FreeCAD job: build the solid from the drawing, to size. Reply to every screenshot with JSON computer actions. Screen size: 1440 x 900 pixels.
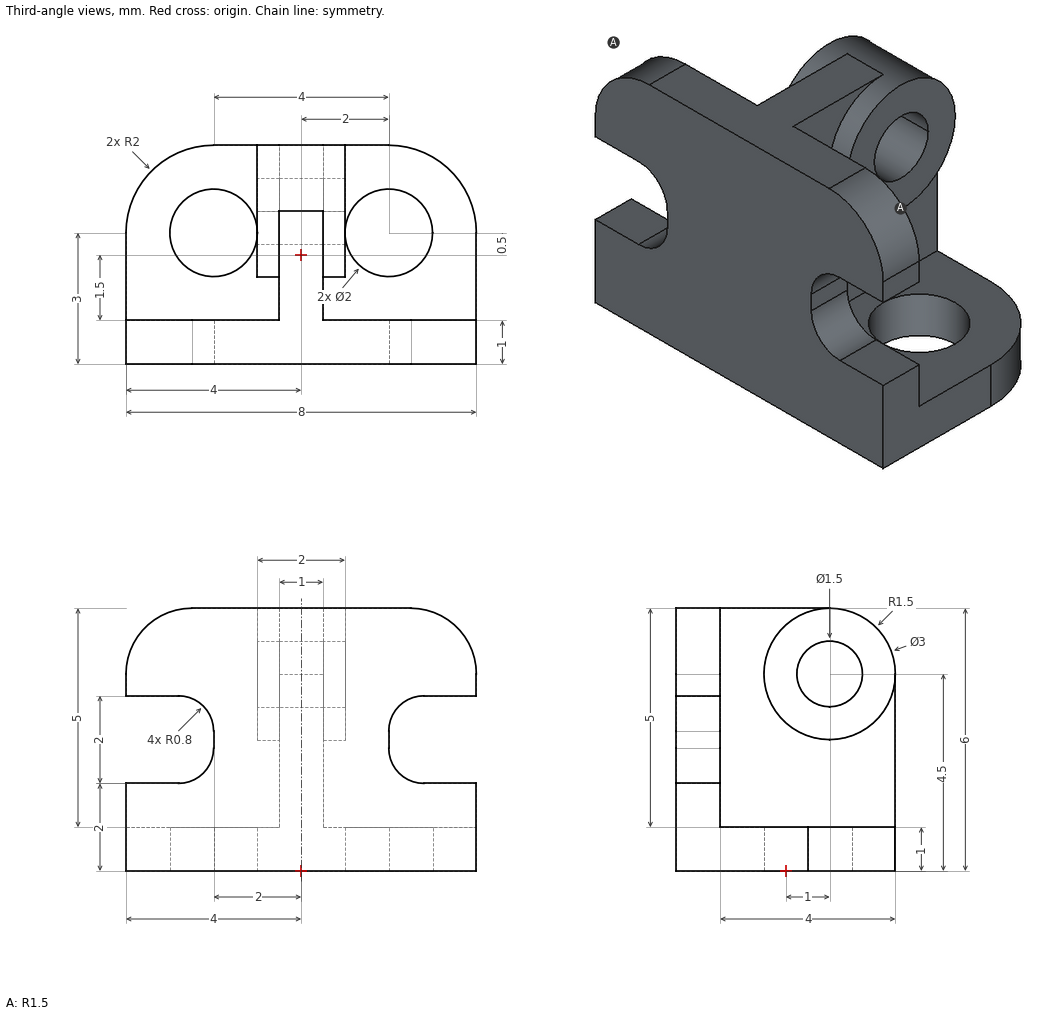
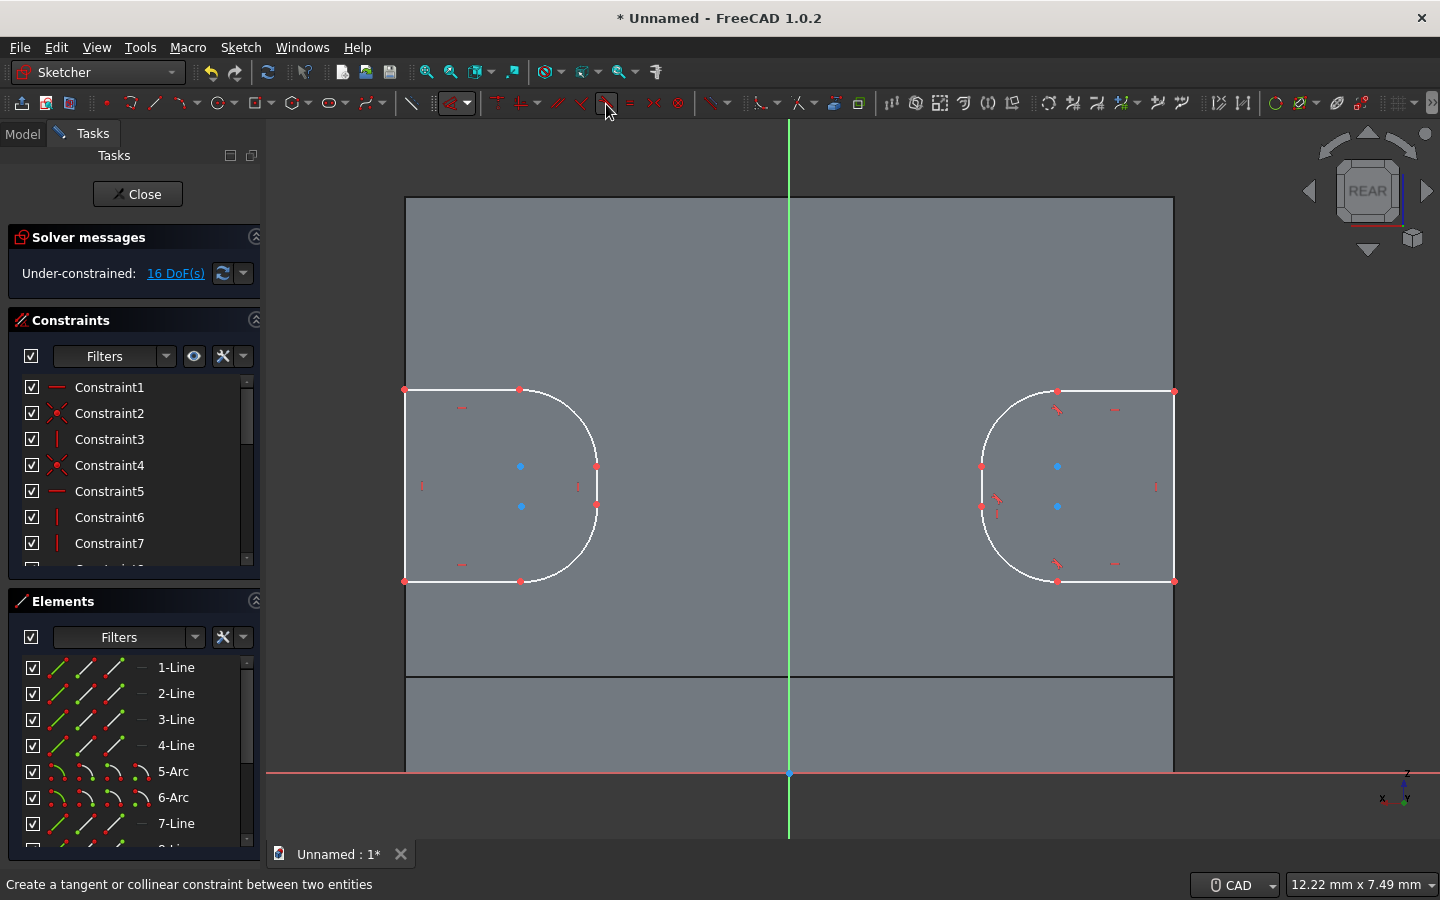
{"action": "left_click", "coordinate": [597, 494]}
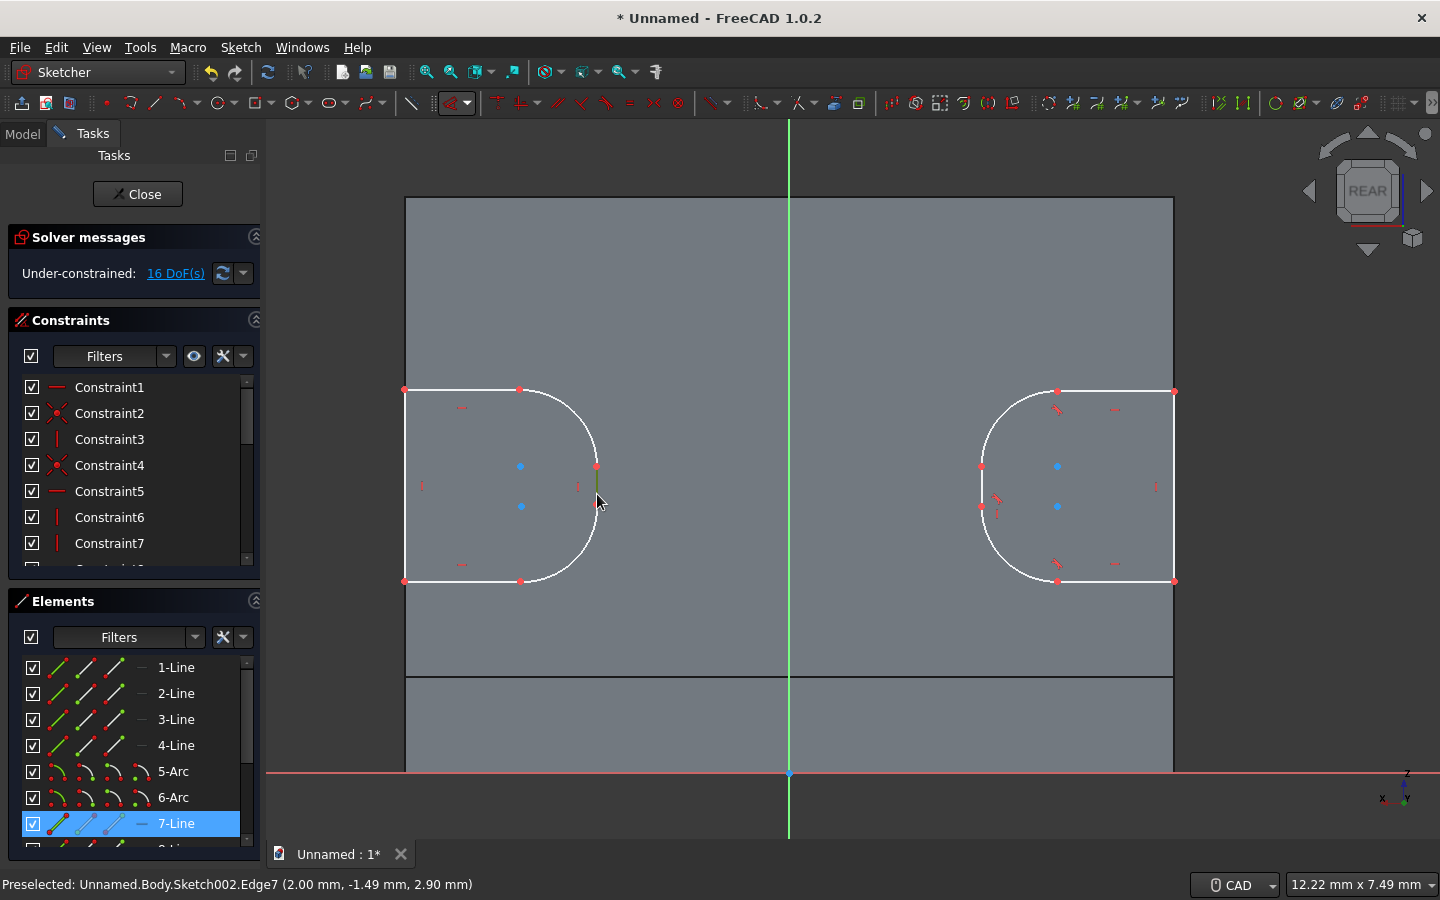
{"action": "left_click", "coordinate": [589, 432]}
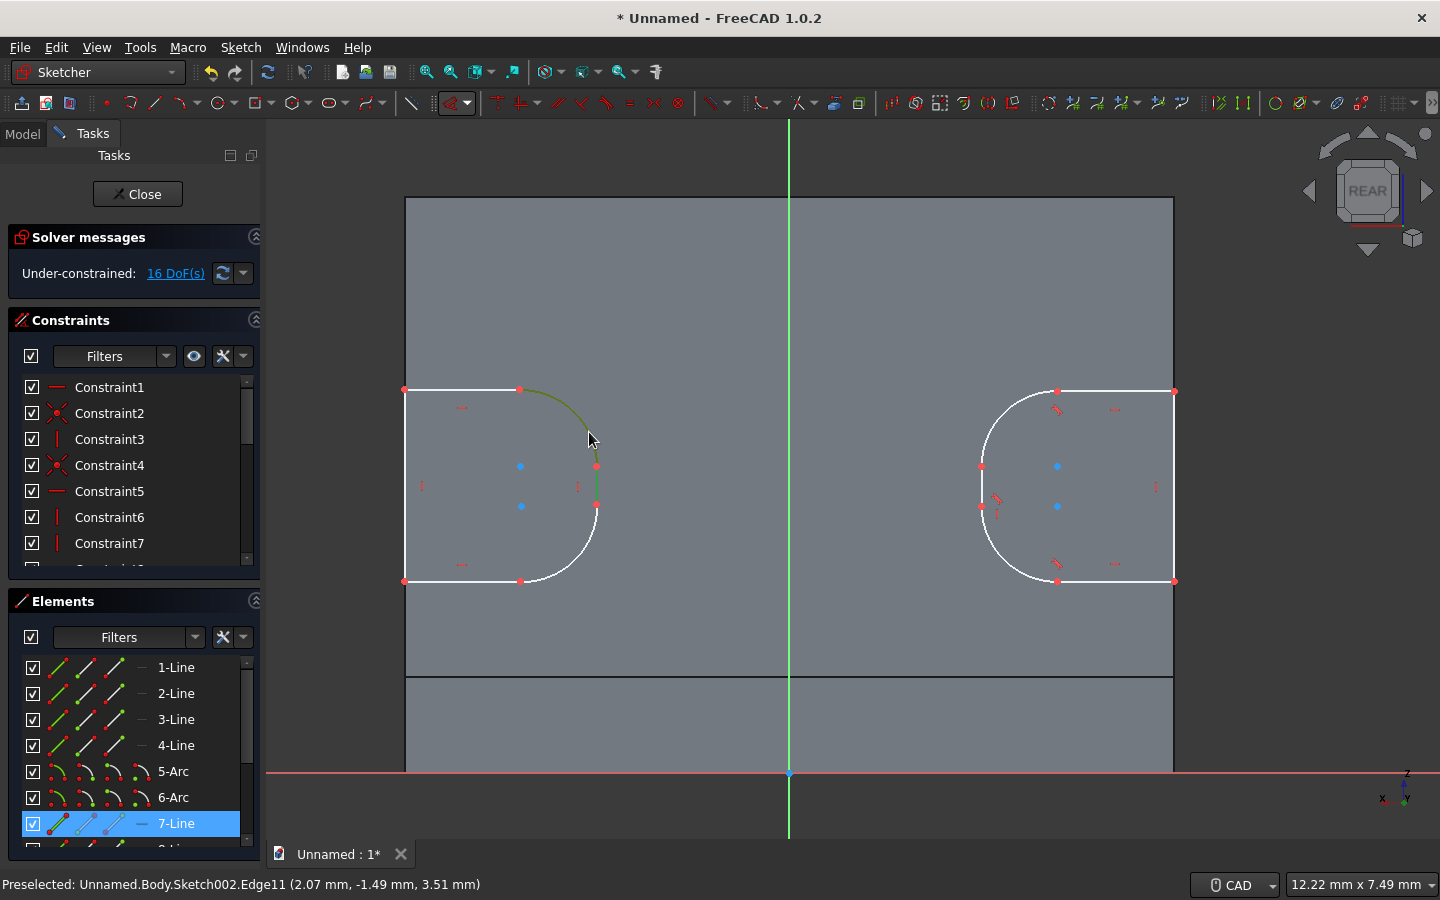
{"action": "left_click", "coordinate": [606, 104]}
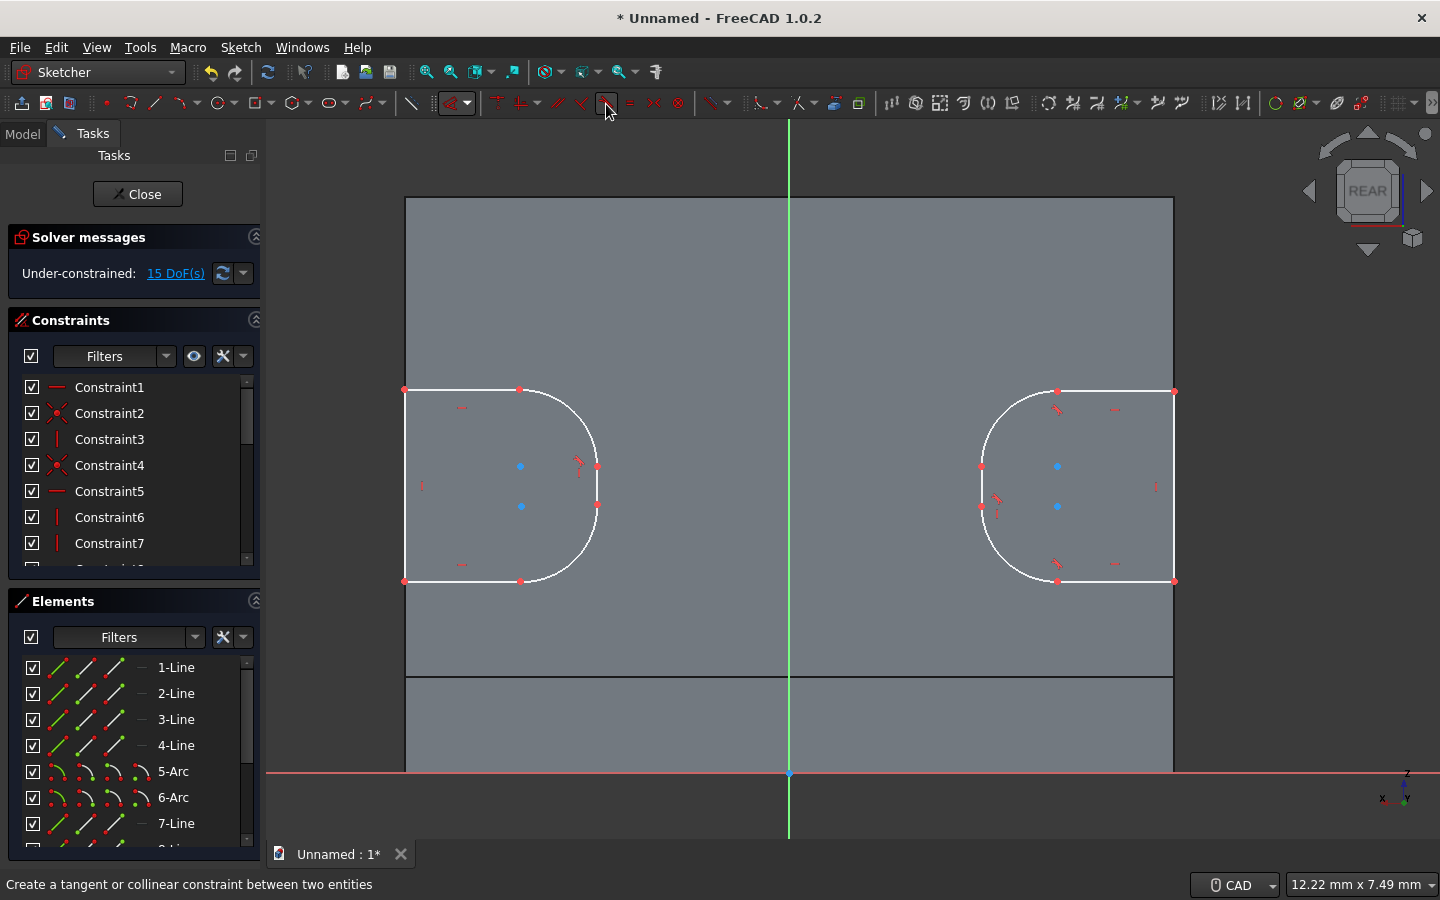
{"action": "left_click", "coordinate": [597, 494]}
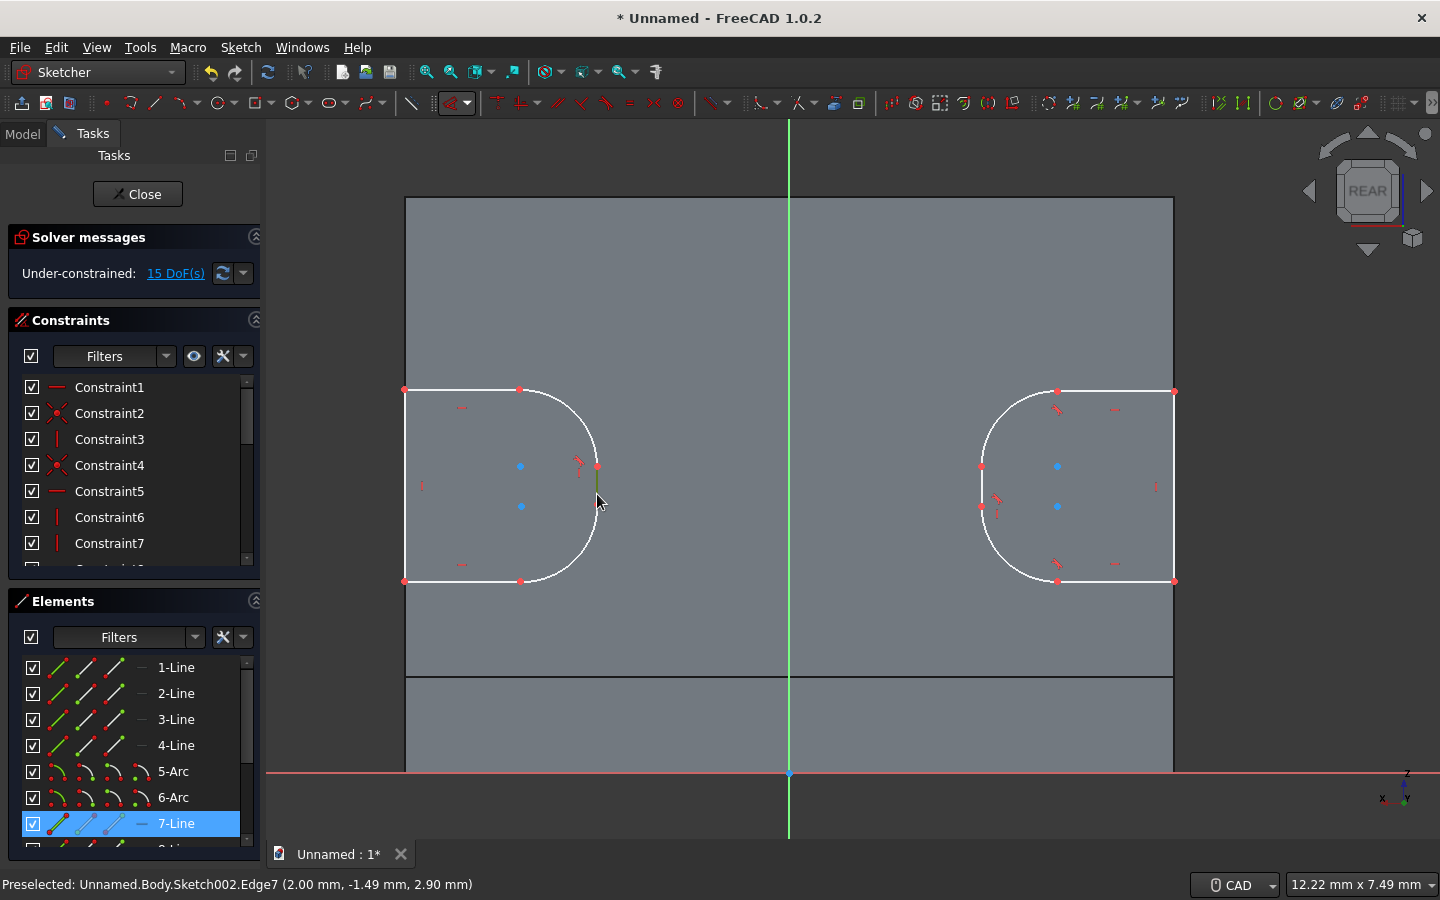
{"action": "left_click", "coordinate": [555, 574]}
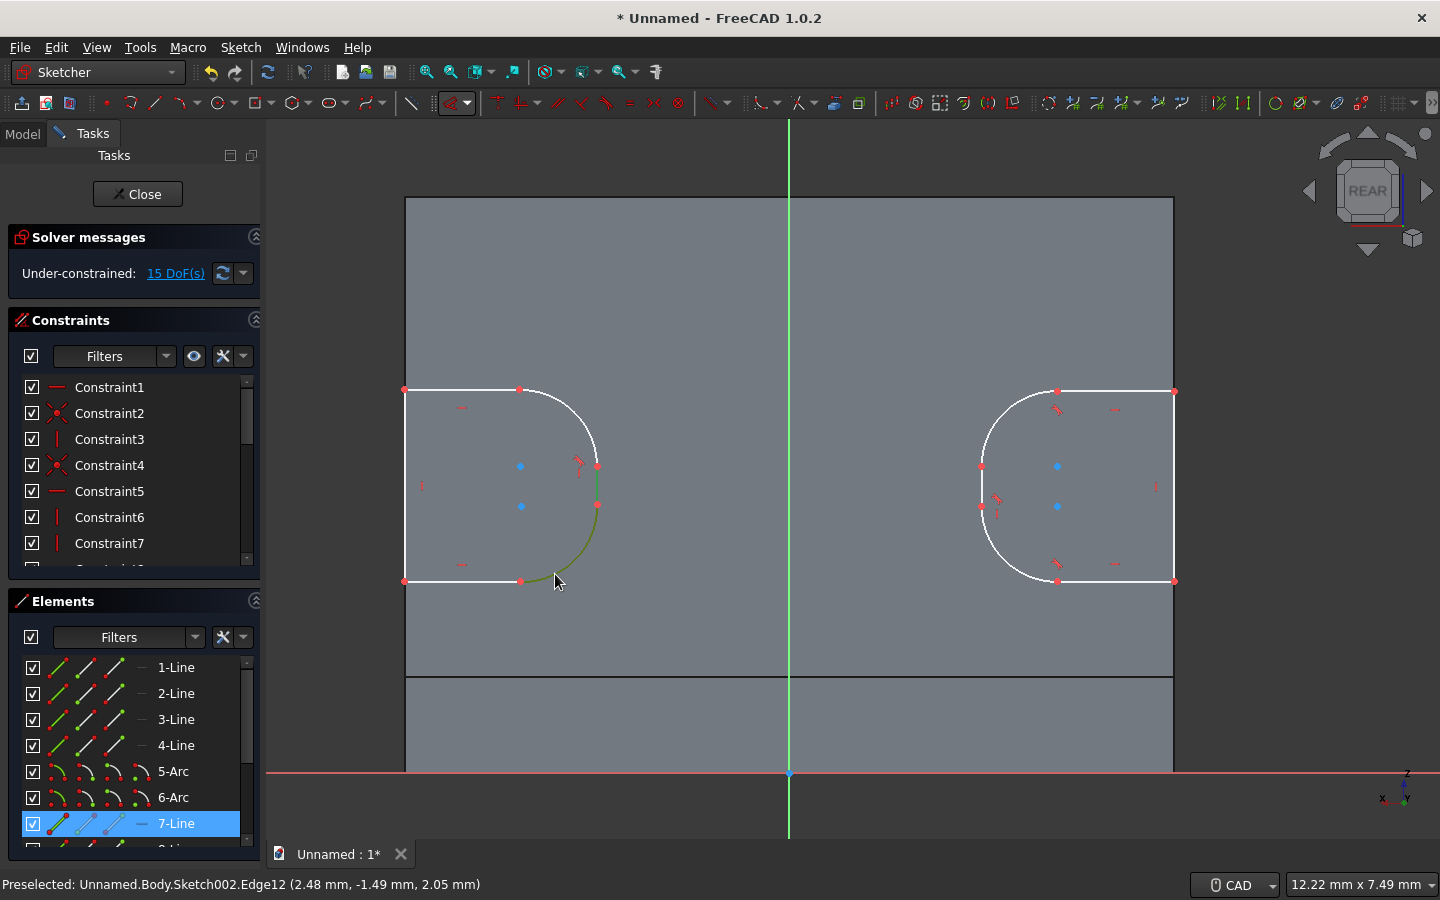
{"action": "left_click", "coordinate": [606, 104]}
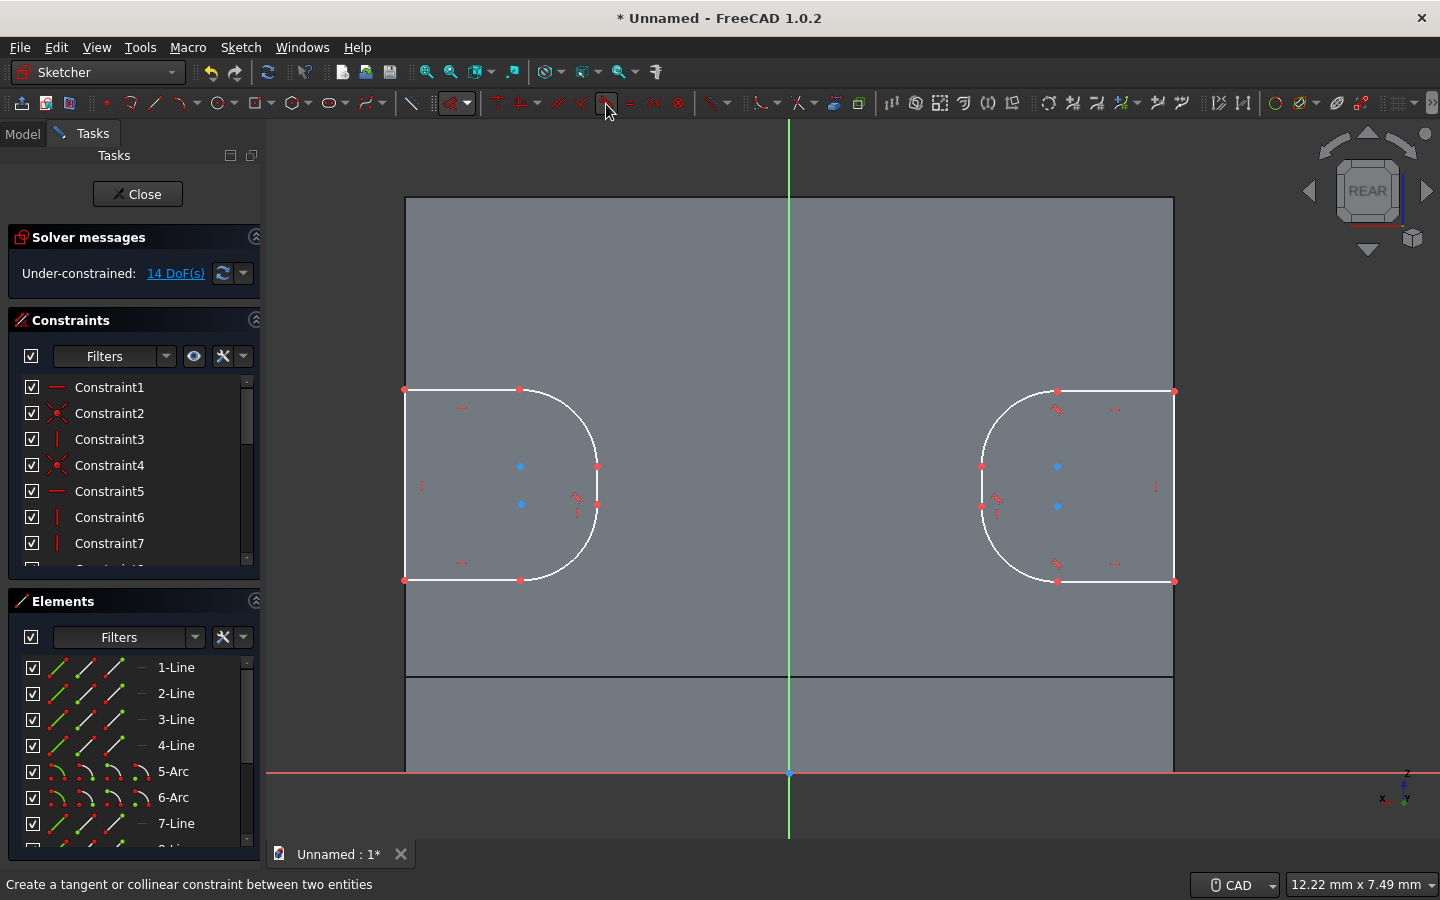
{"action": "left_click", "coordinate": [485, 390]}